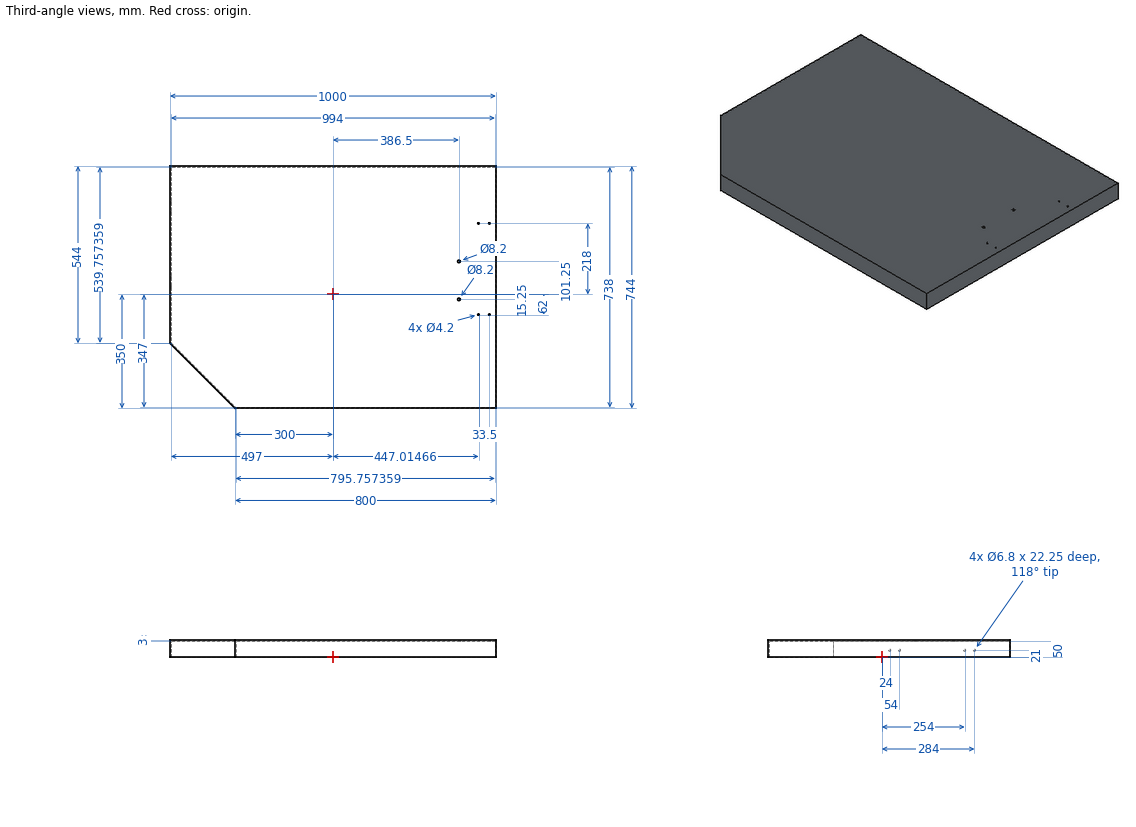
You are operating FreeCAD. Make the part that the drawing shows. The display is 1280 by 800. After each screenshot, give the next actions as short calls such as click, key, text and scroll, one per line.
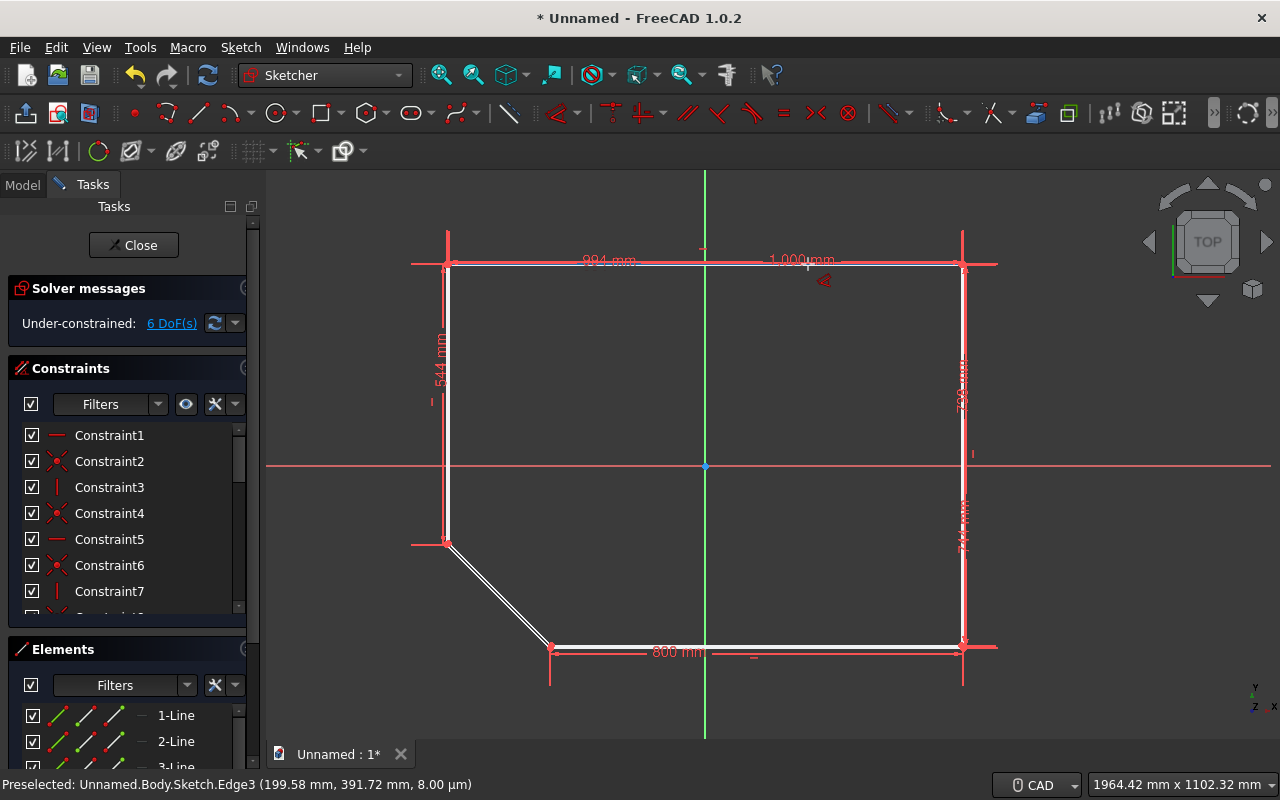
scroll(550, 648, up, 8)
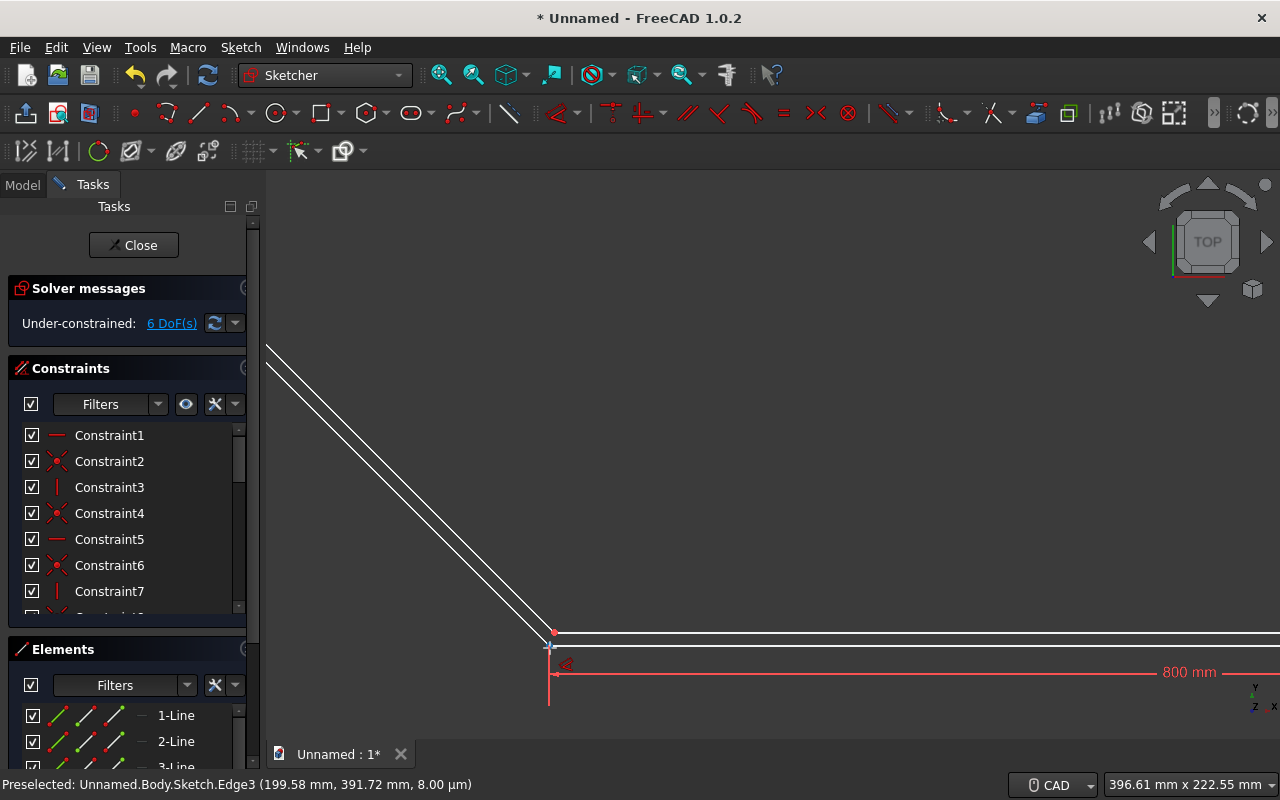
click(549, 646)
click(832, 680)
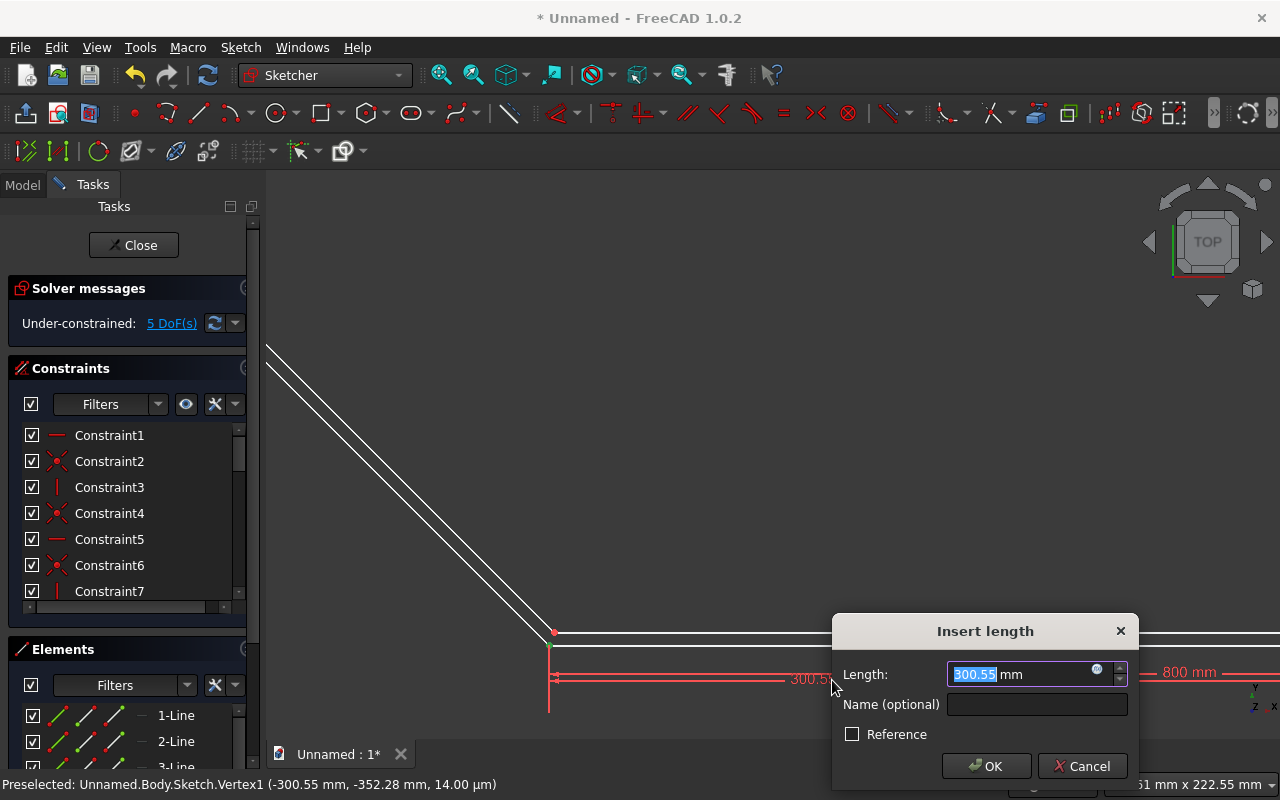
text(300)
key(Return)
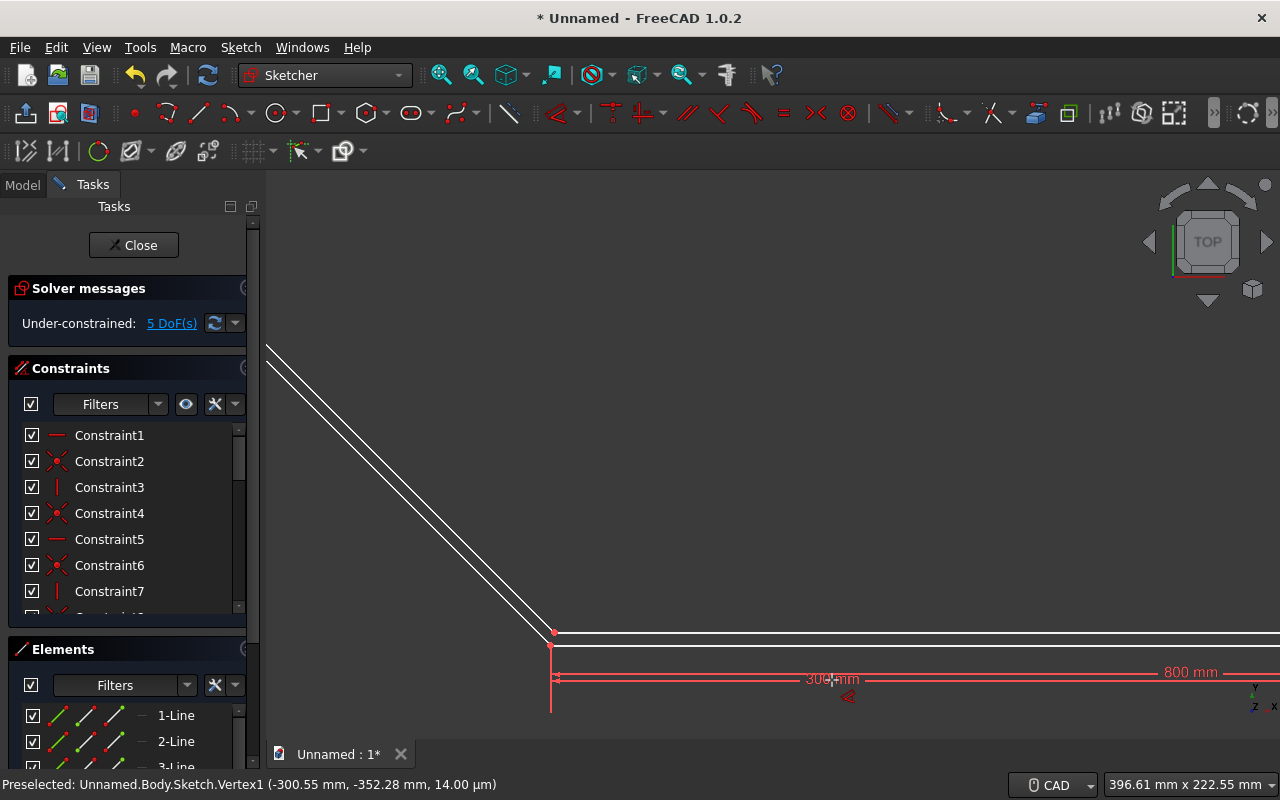
click(551, 646)
click(517, 422)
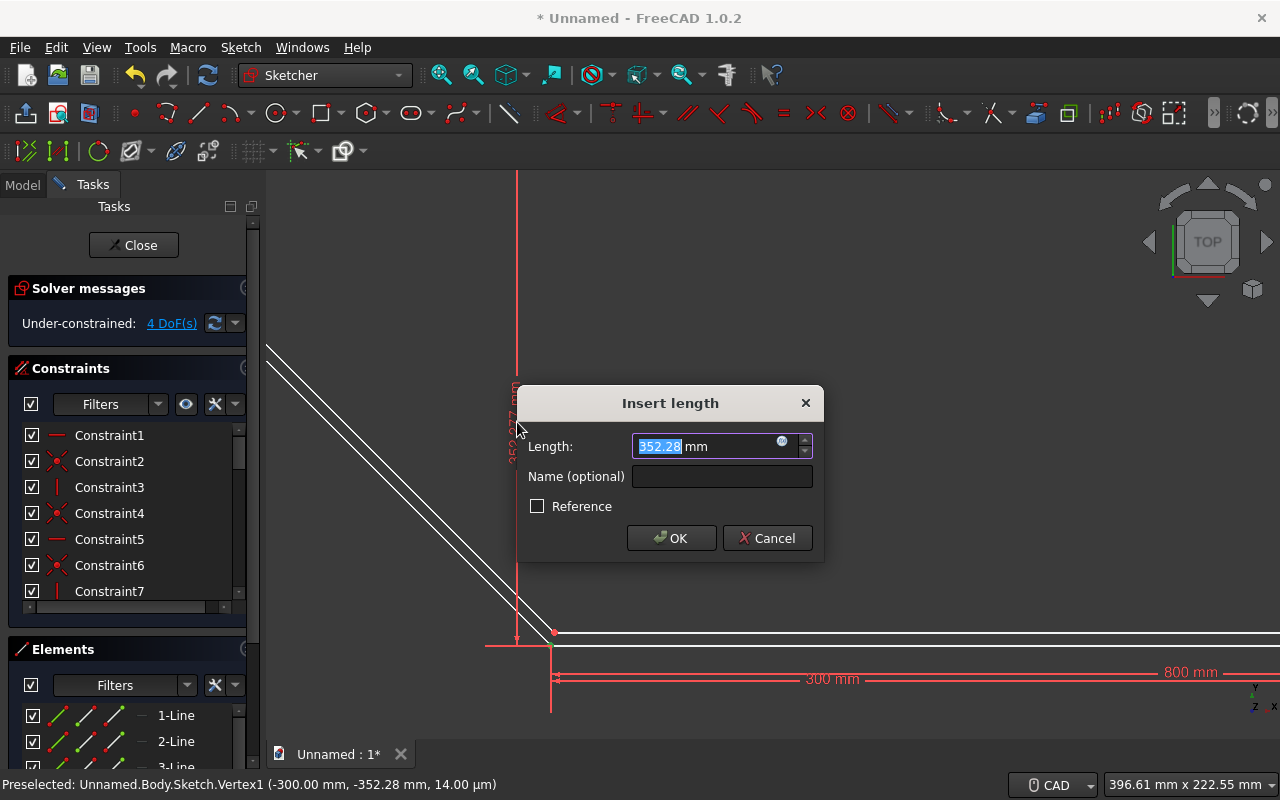
text(350)
key(Return)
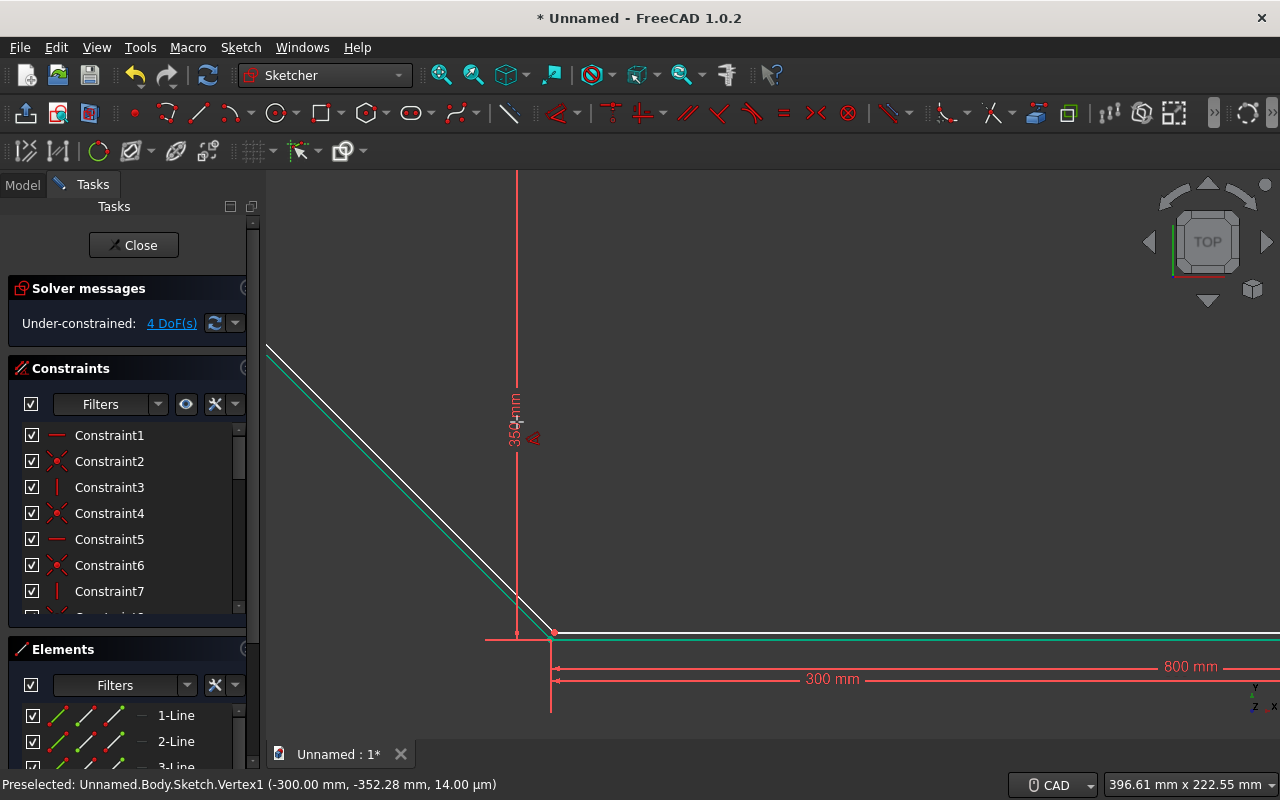
scroll(554, 633, up, 3)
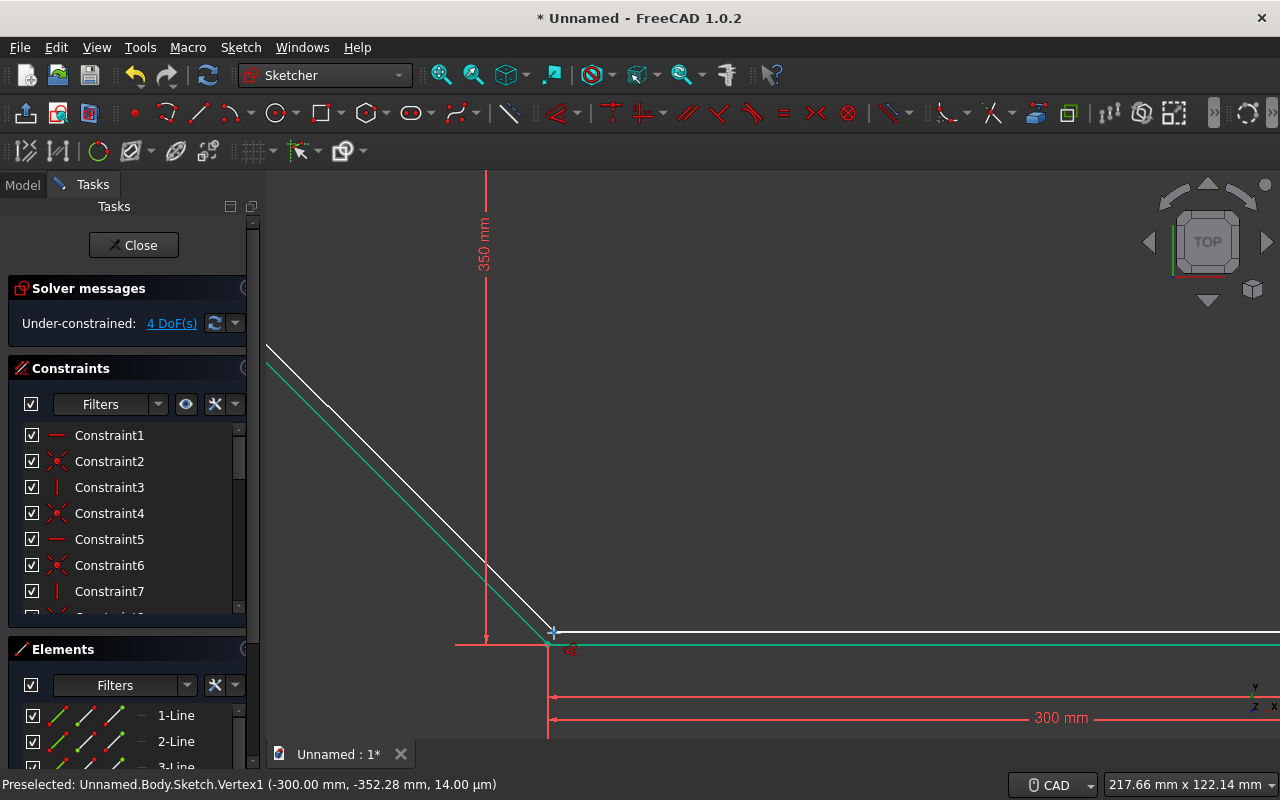
click(554, 632)
click(520, 415)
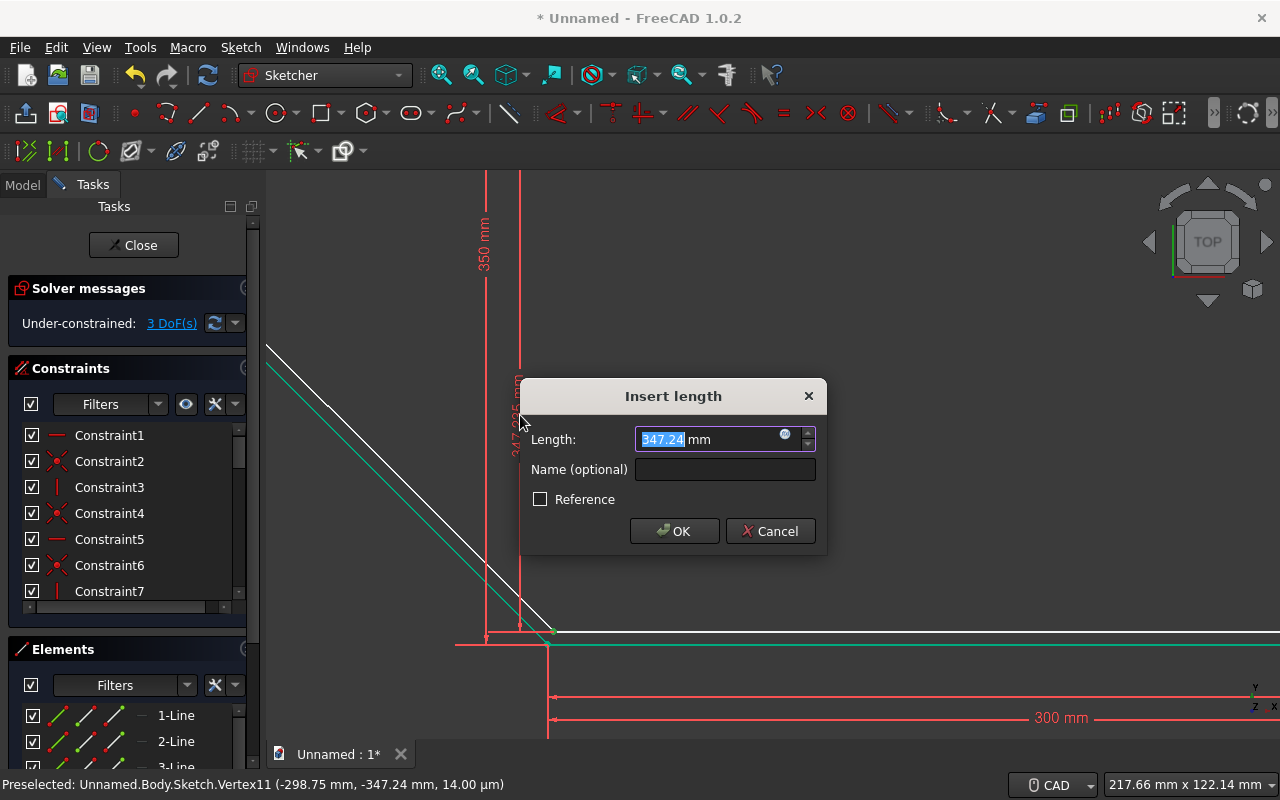
text(347)
key(Return)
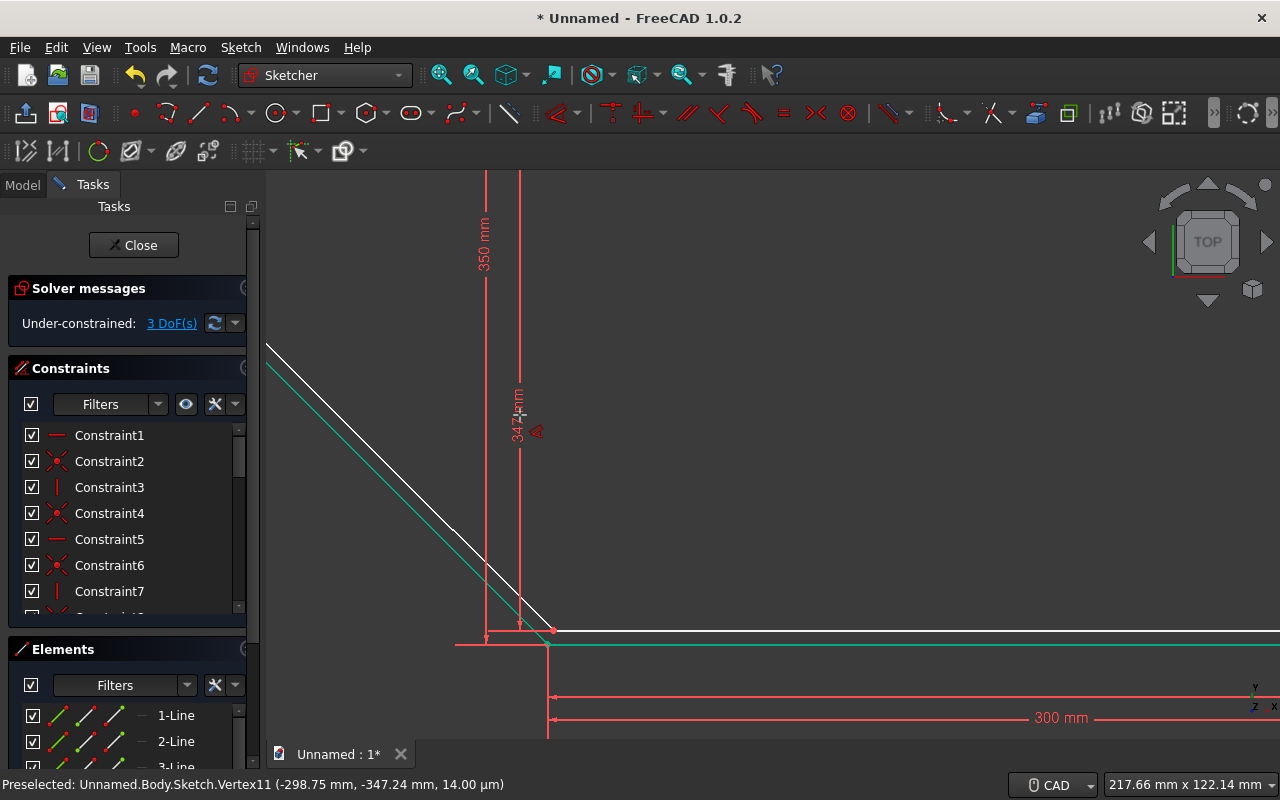
scroll(550, 647, down, 11)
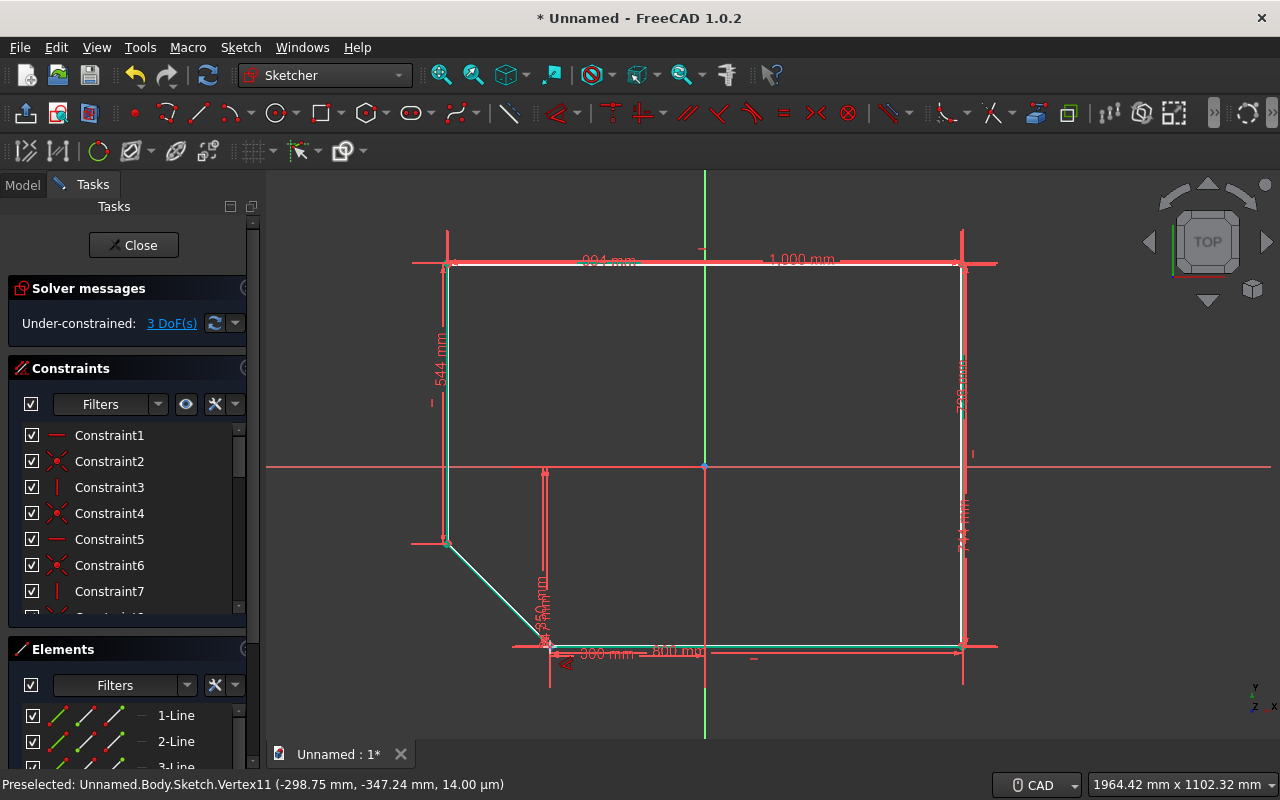
scroll(448, 544, up, 11)